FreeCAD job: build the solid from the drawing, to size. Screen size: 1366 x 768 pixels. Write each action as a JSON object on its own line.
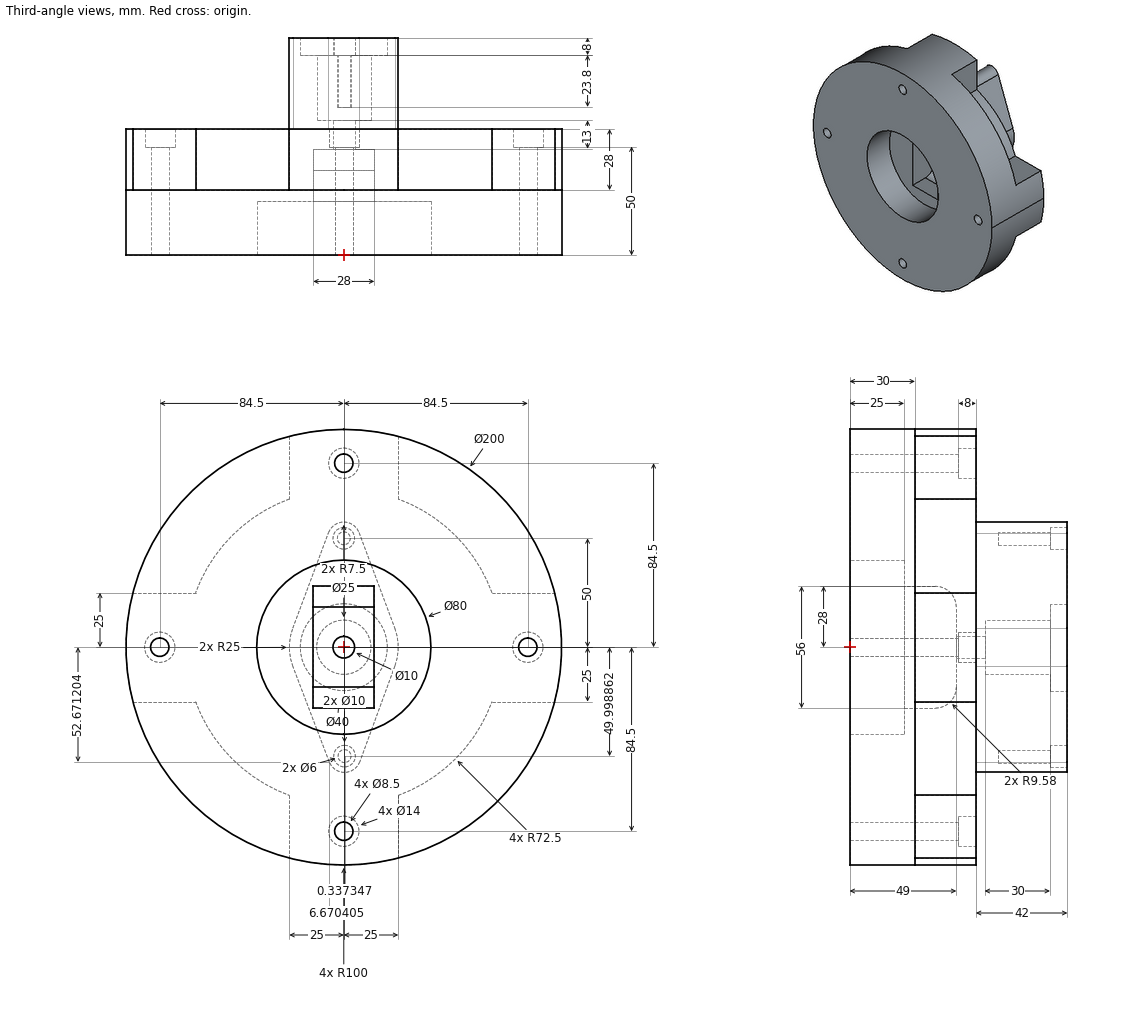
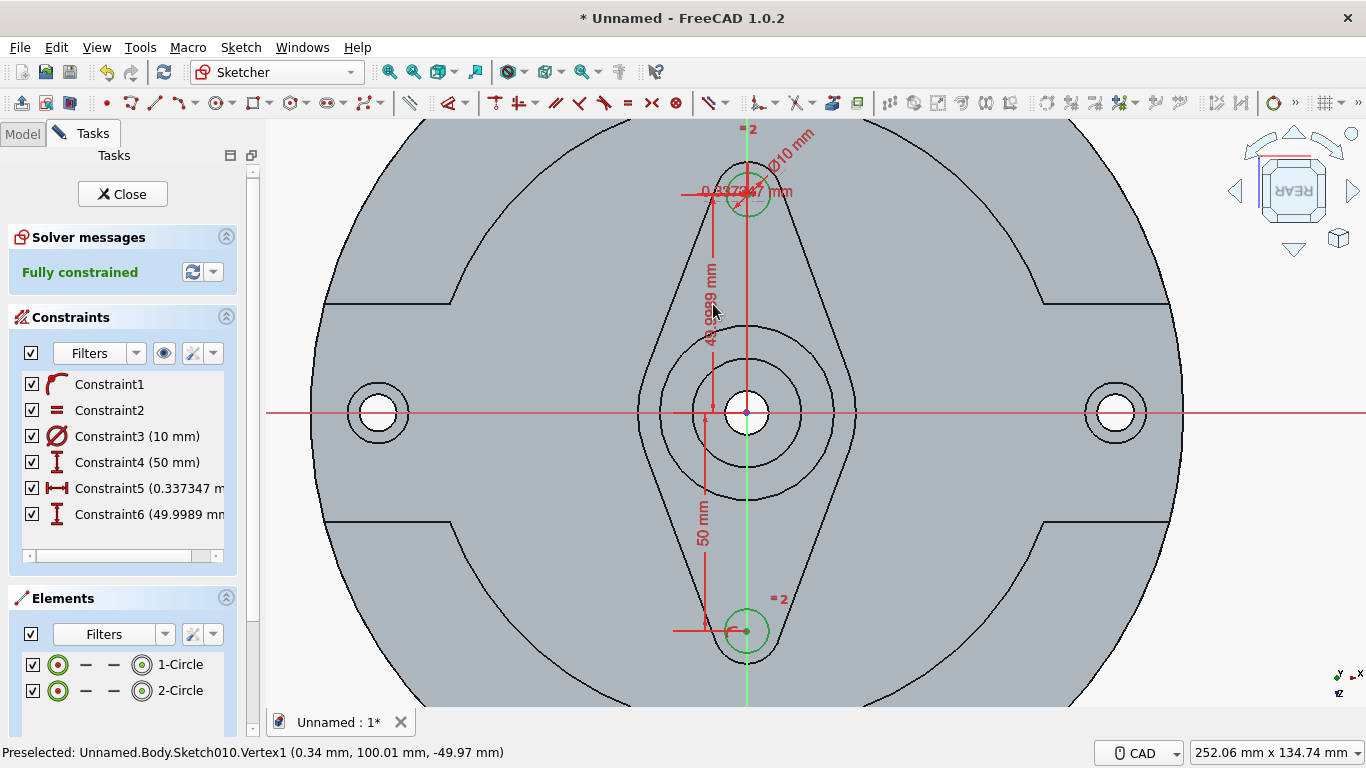
{"action": "left_click", "coordinate": [123, 194]}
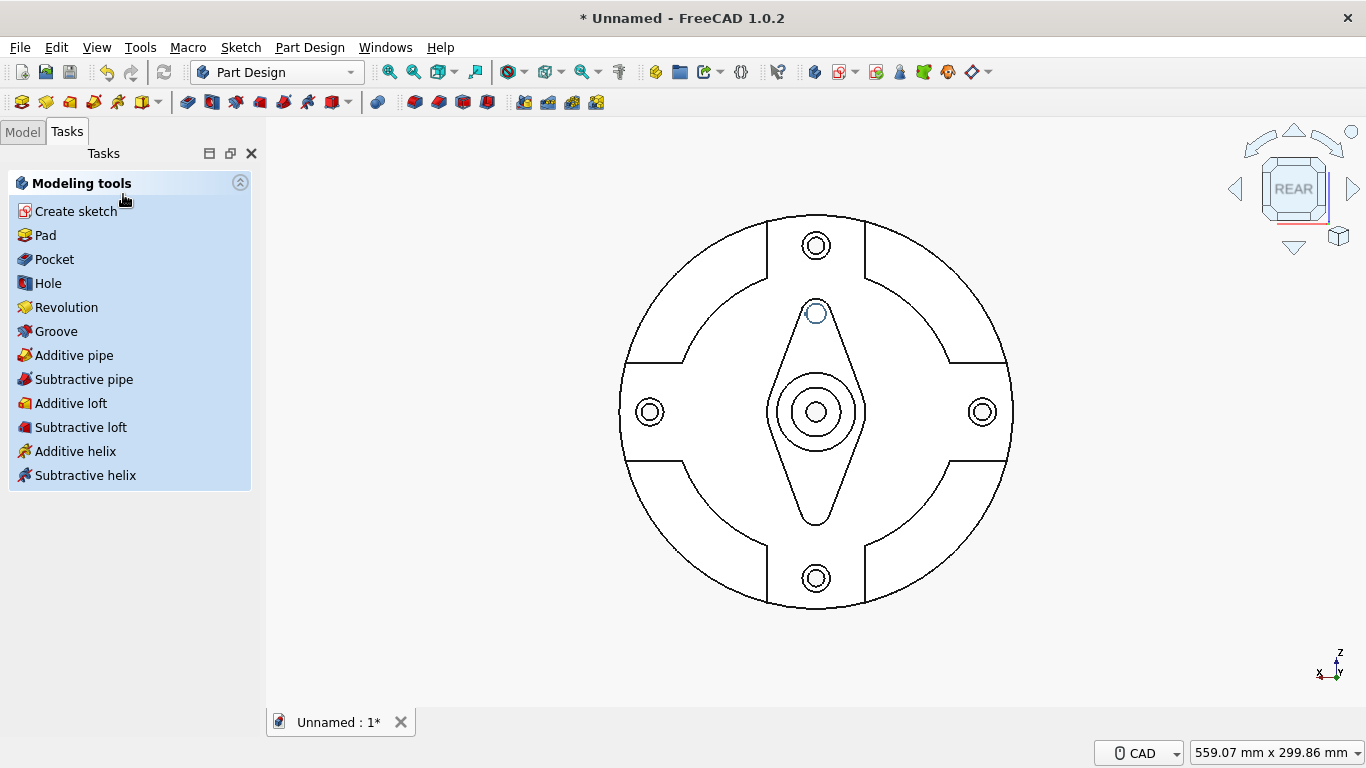
{"action": "left_click", "coordinate": [188, 102]}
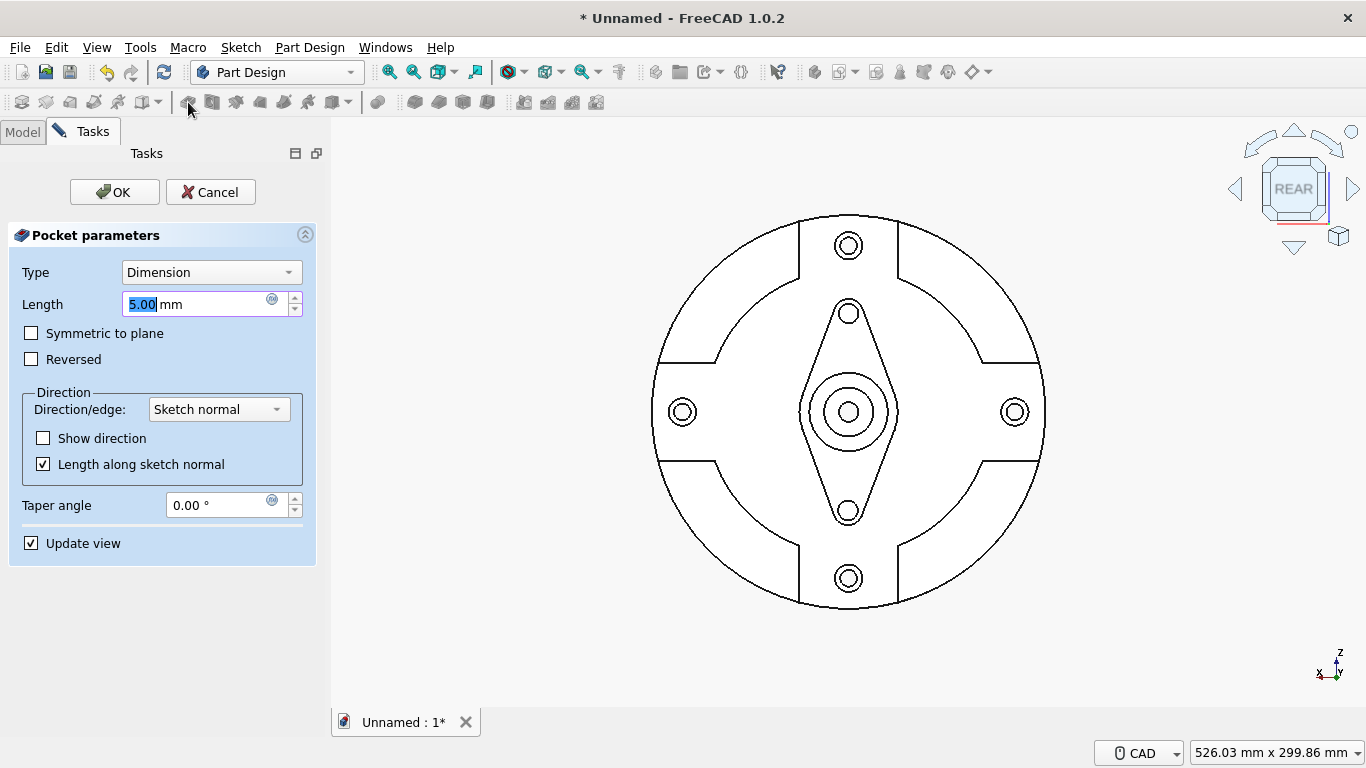
{"action": "type", "text": "8"}
{"action": "key", "text": "Tab"}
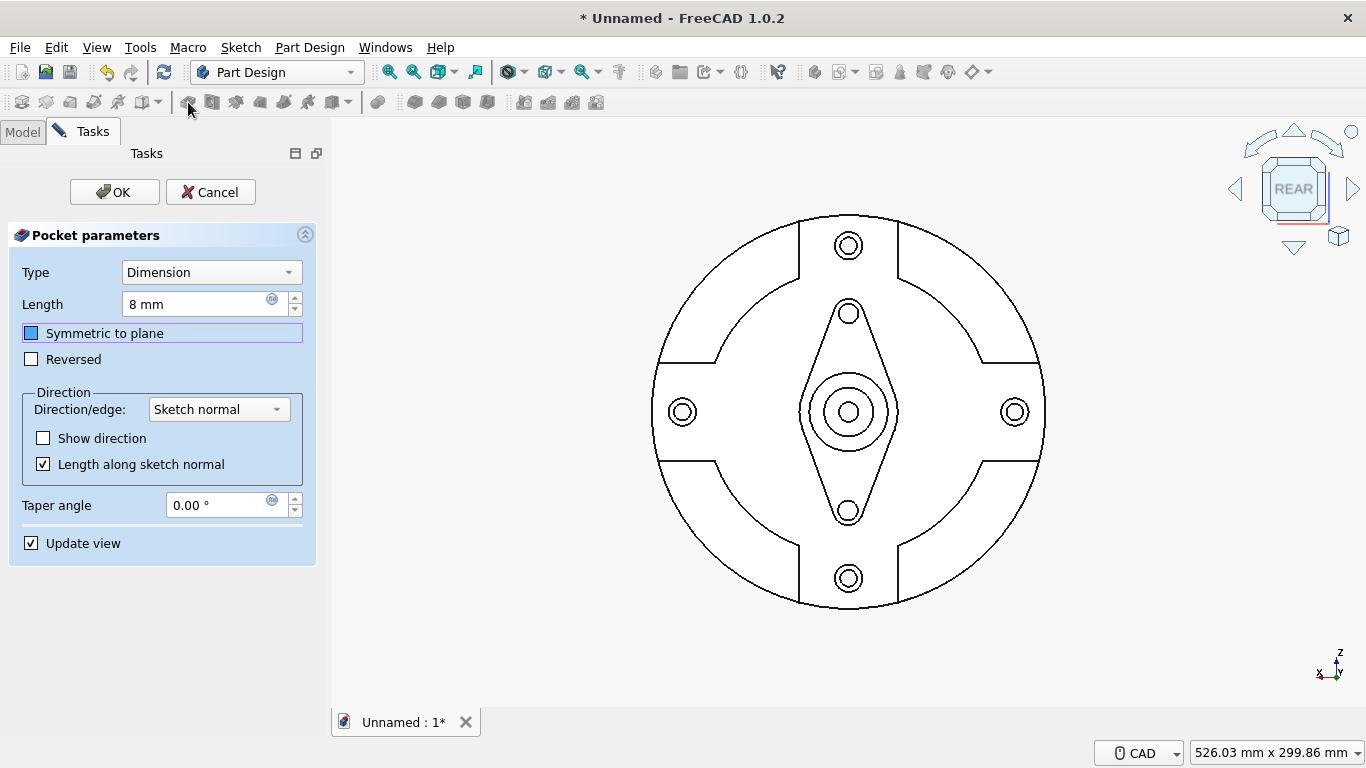
{"action": "left_click", "coordinate": [115, 192]}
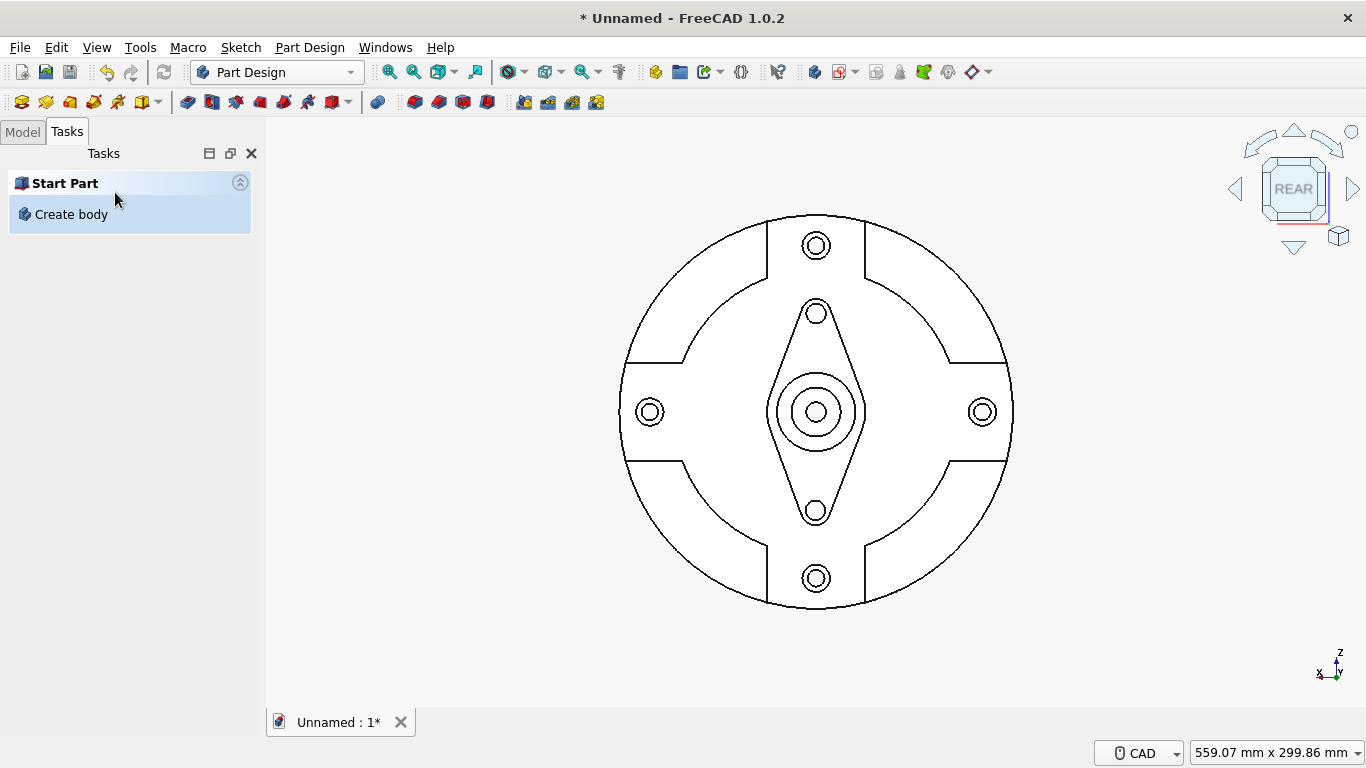
{"action": "key", "text": "5"}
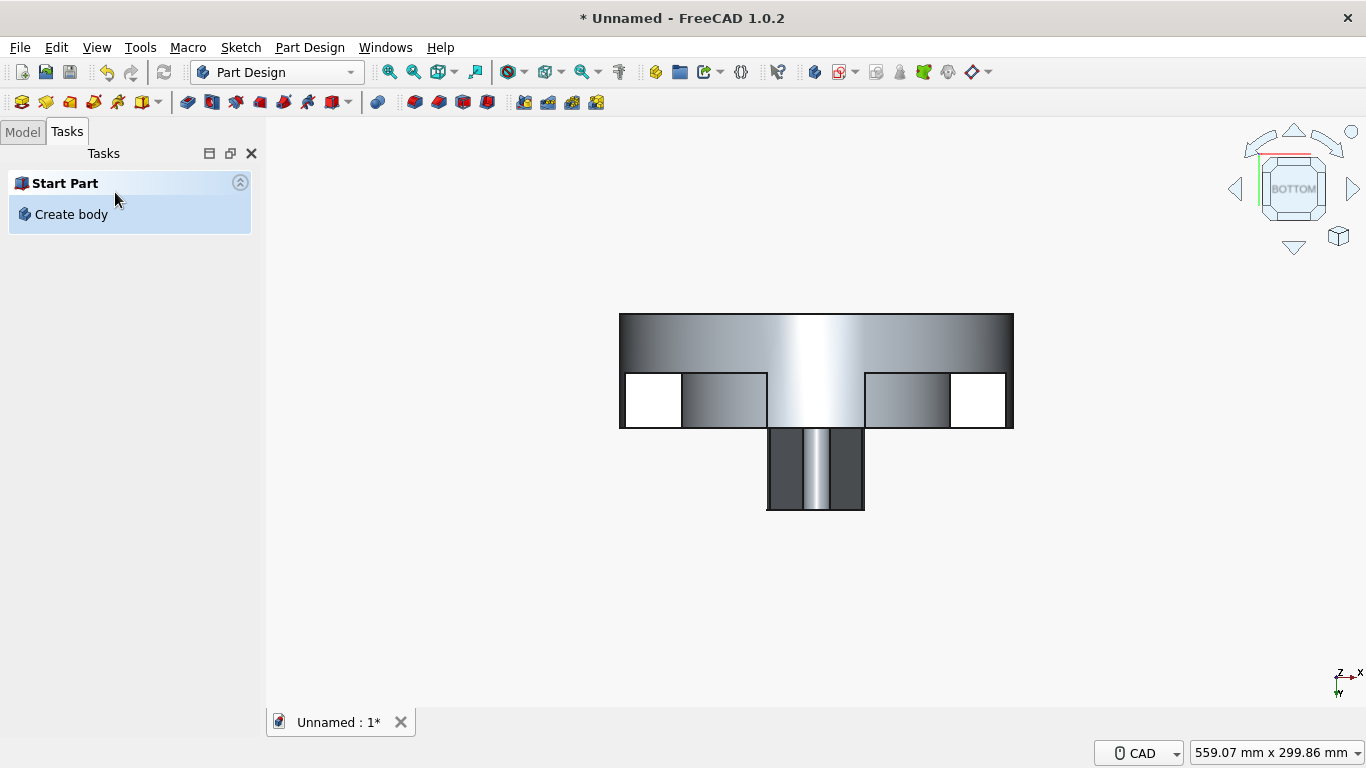
{"action": "key", "text": "v f"}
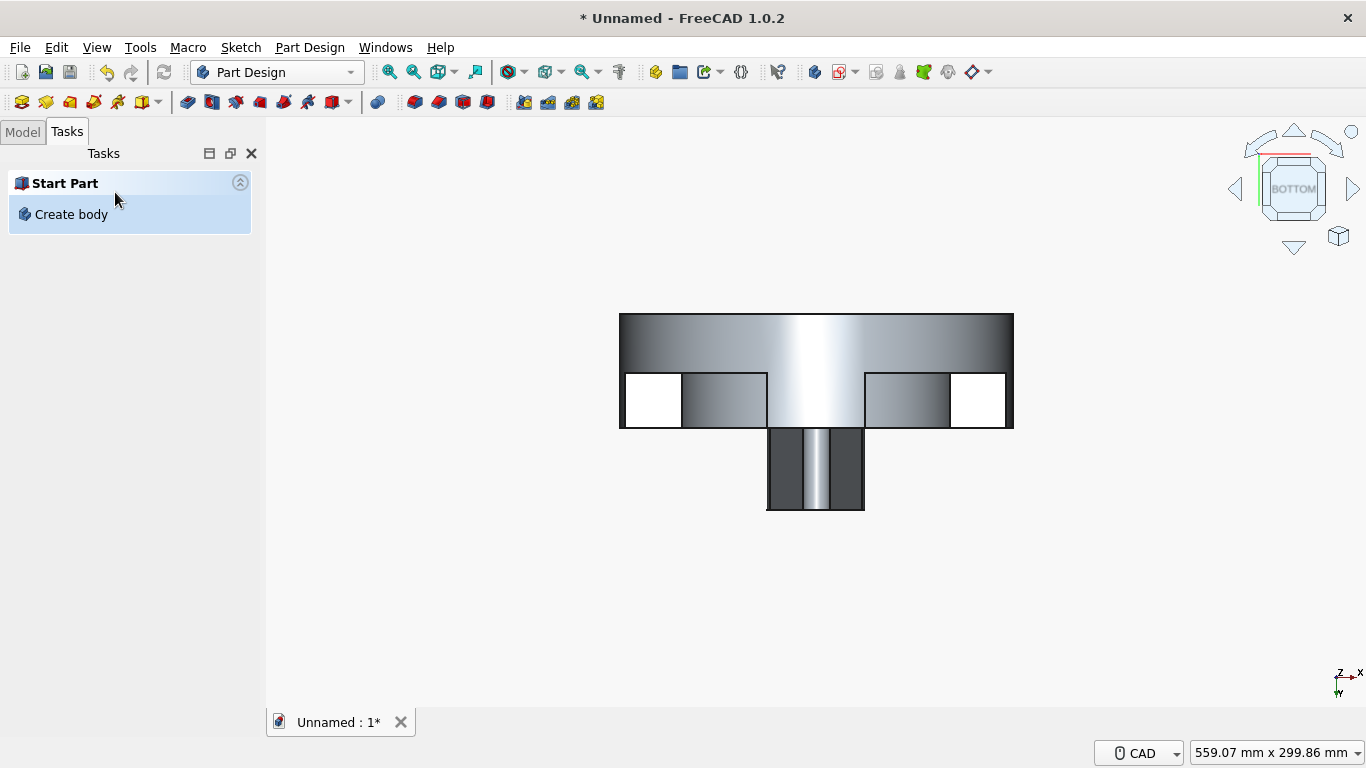
{"action": "key", "text": "4"}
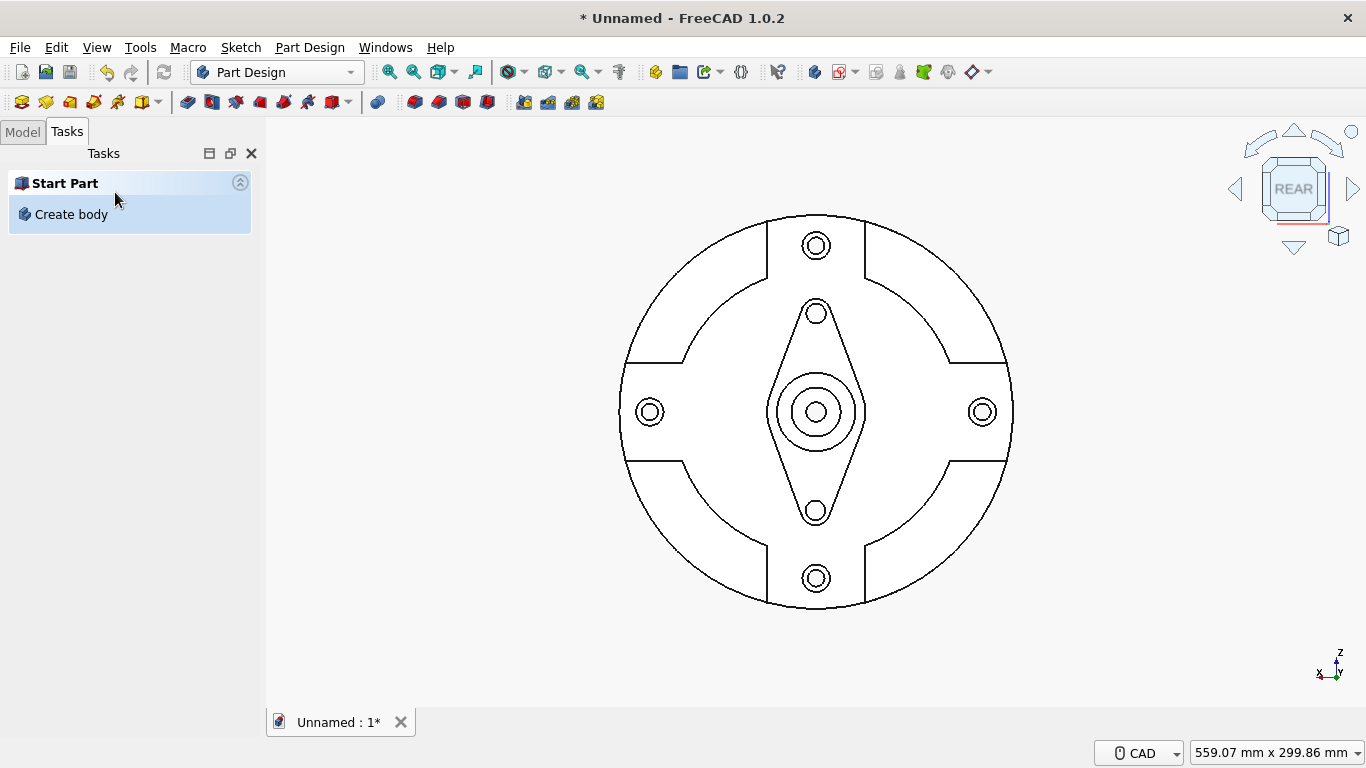
{"action": "key", "text": "3"}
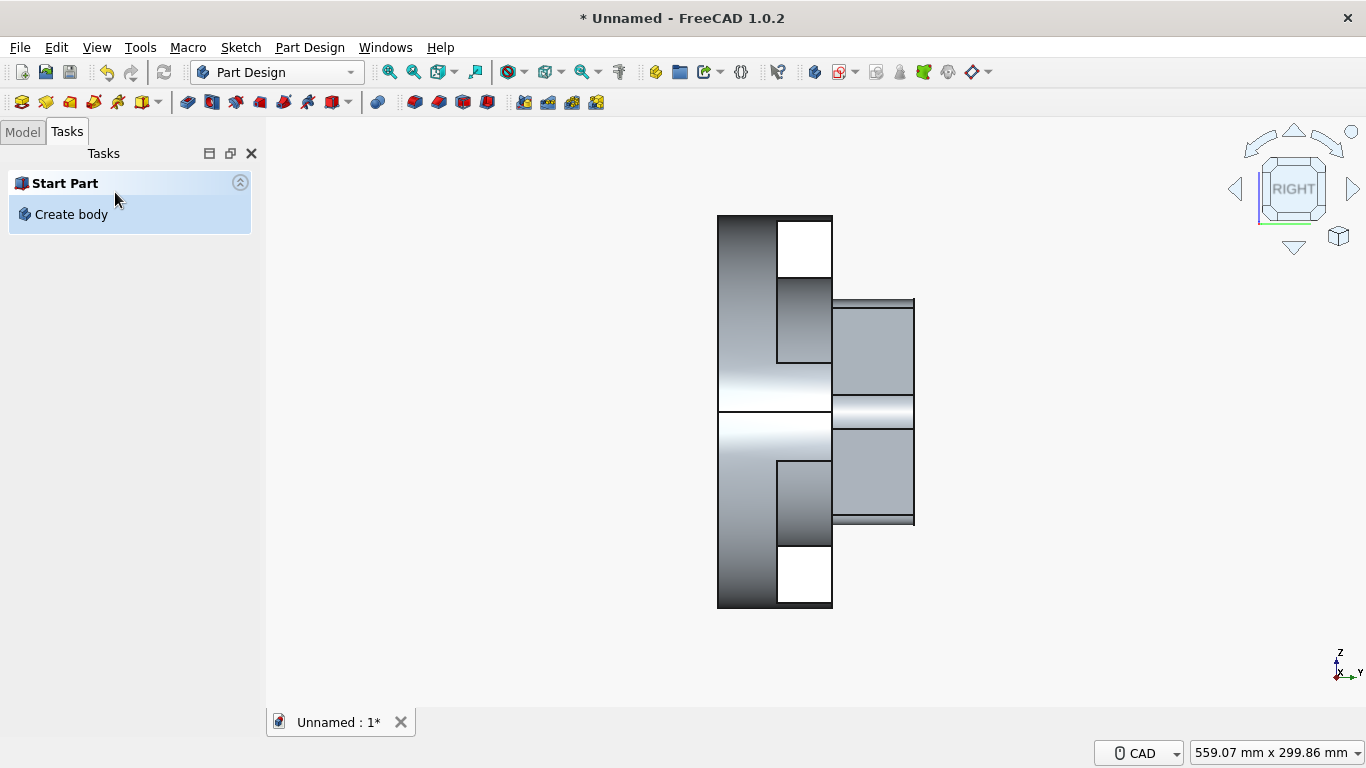
{"action": "left_click", "coordinate": [23, 131]}